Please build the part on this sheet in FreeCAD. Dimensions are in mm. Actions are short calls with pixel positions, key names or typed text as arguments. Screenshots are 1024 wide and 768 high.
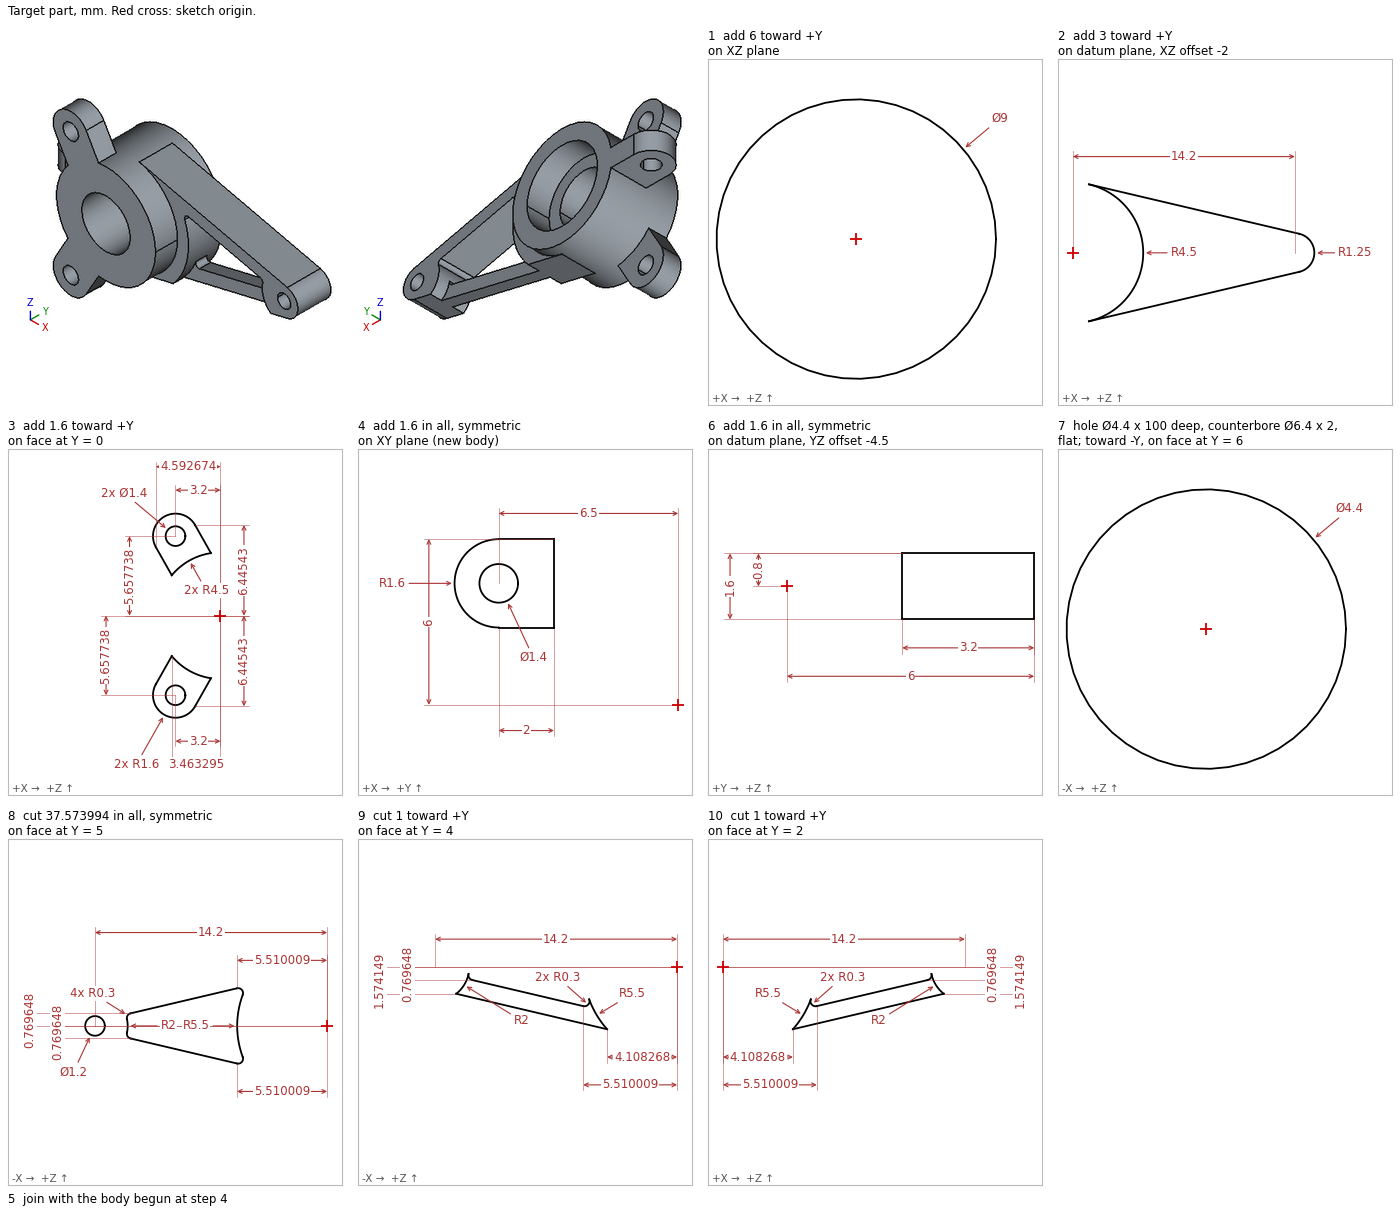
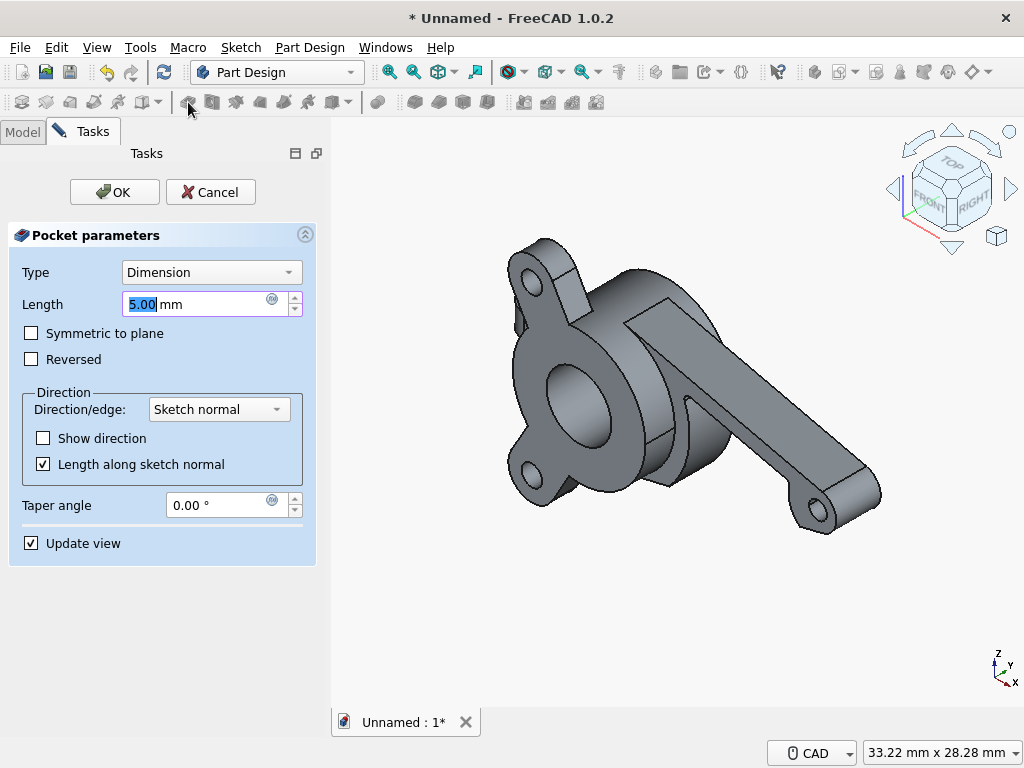
text(1)
key(Tab)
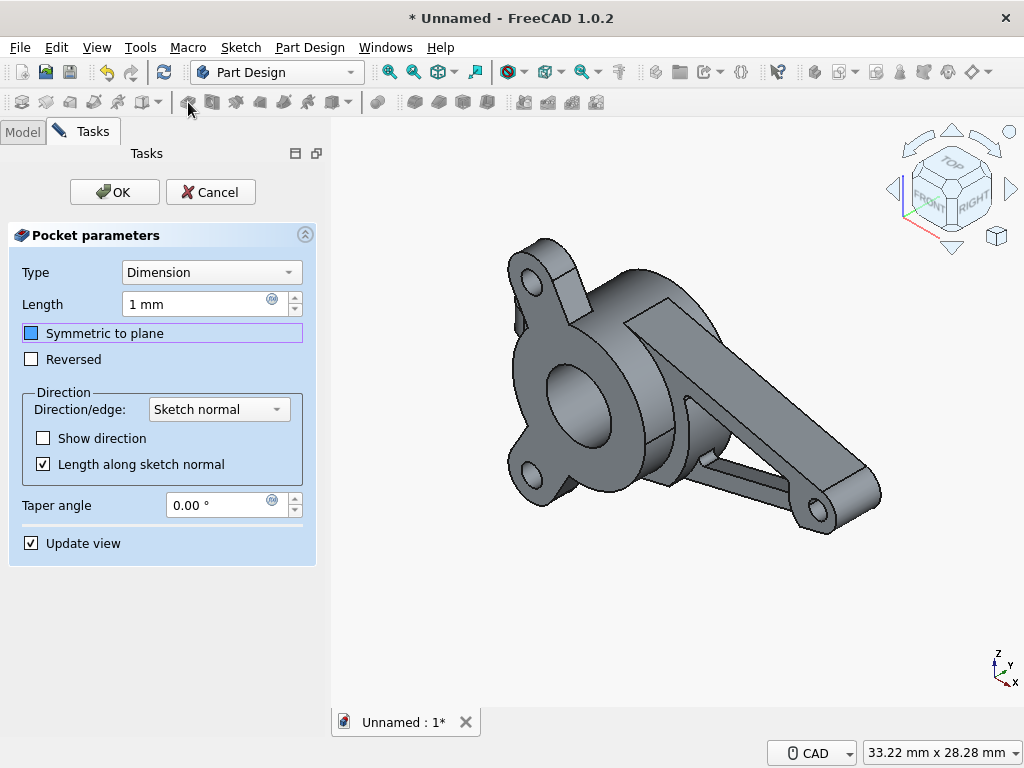
click(115, 192)